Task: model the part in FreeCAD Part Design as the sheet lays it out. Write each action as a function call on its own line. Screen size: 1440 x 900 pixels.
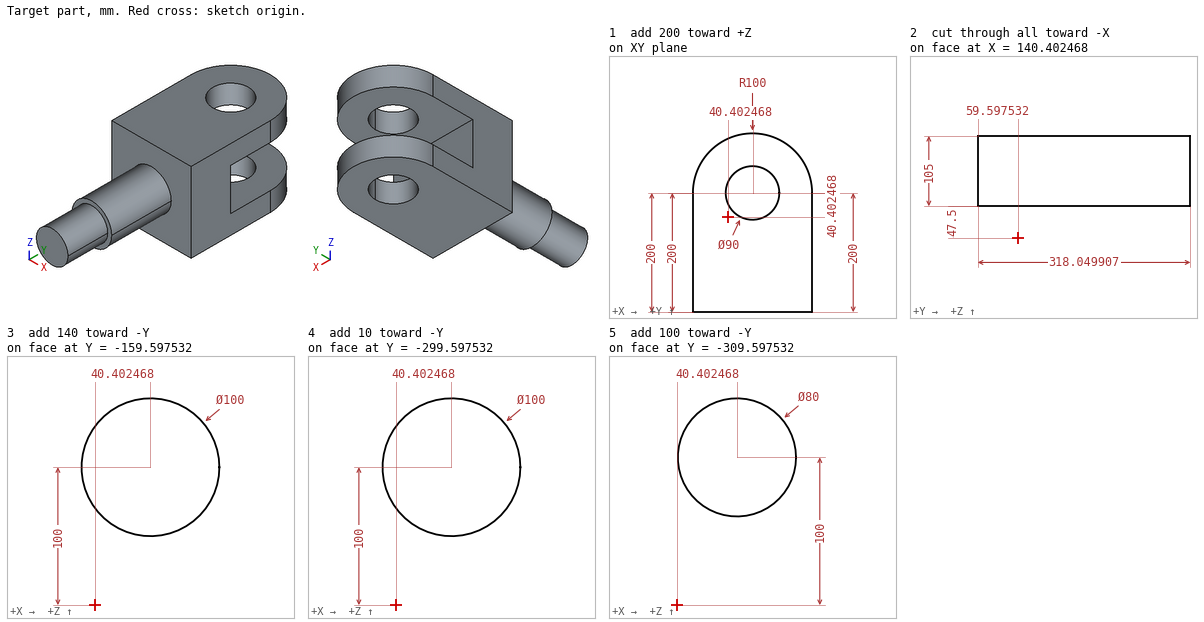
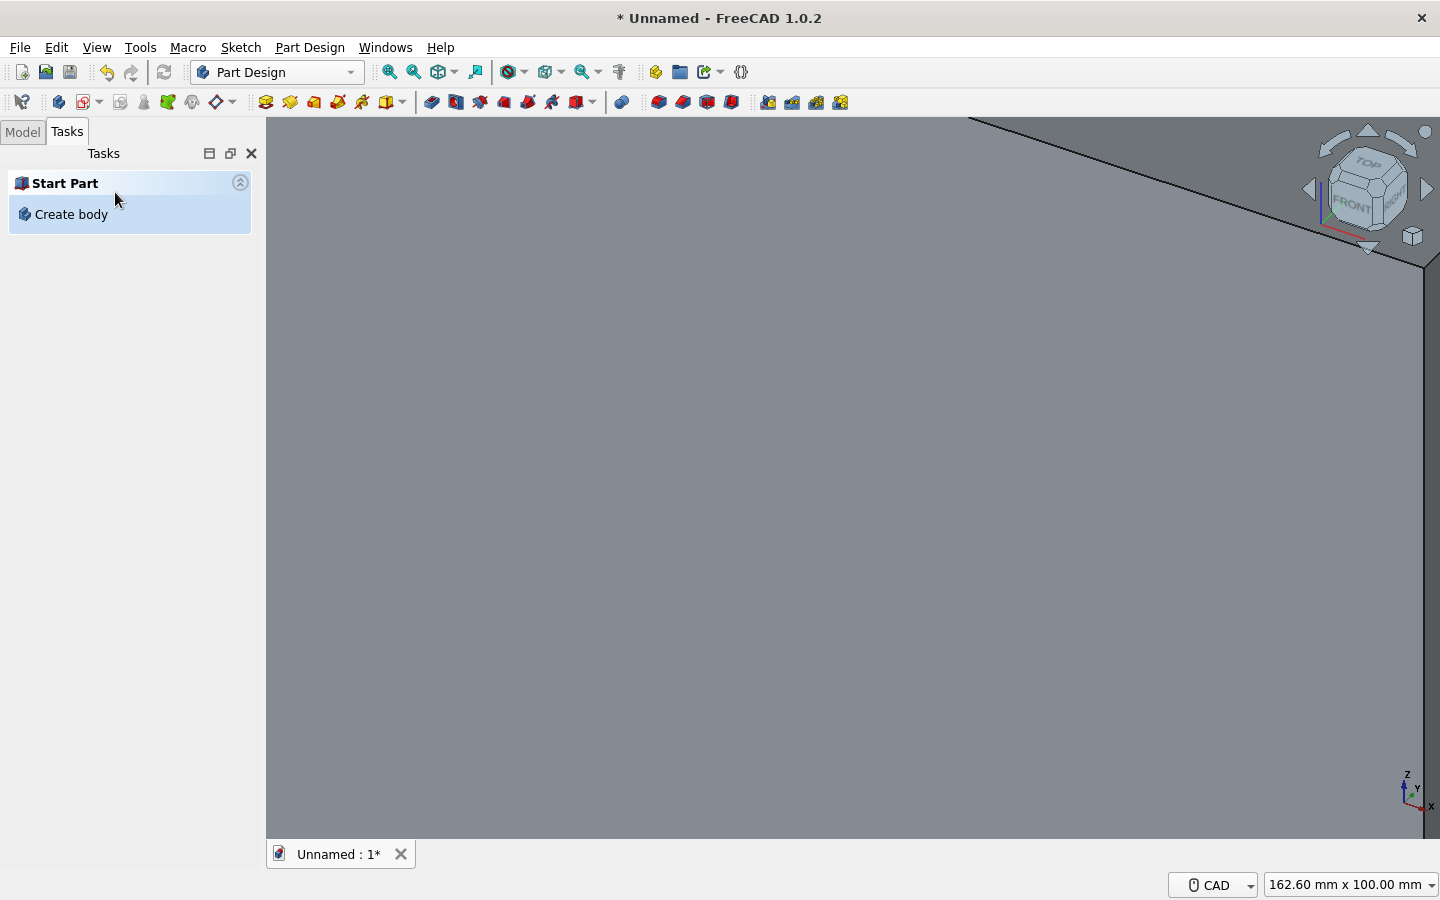
key(v)
key(f)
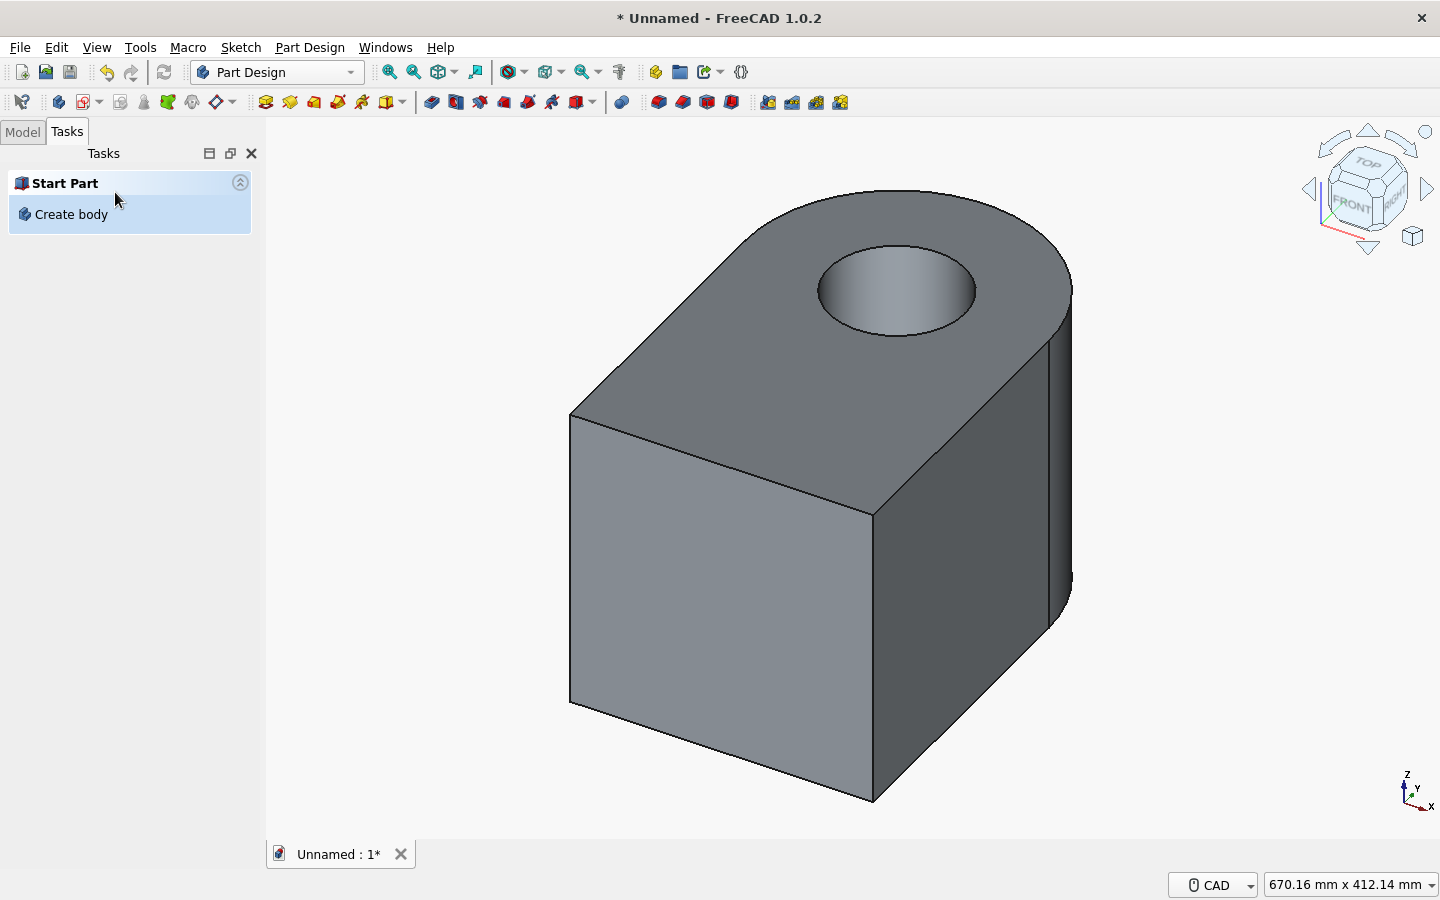
click(961, 571)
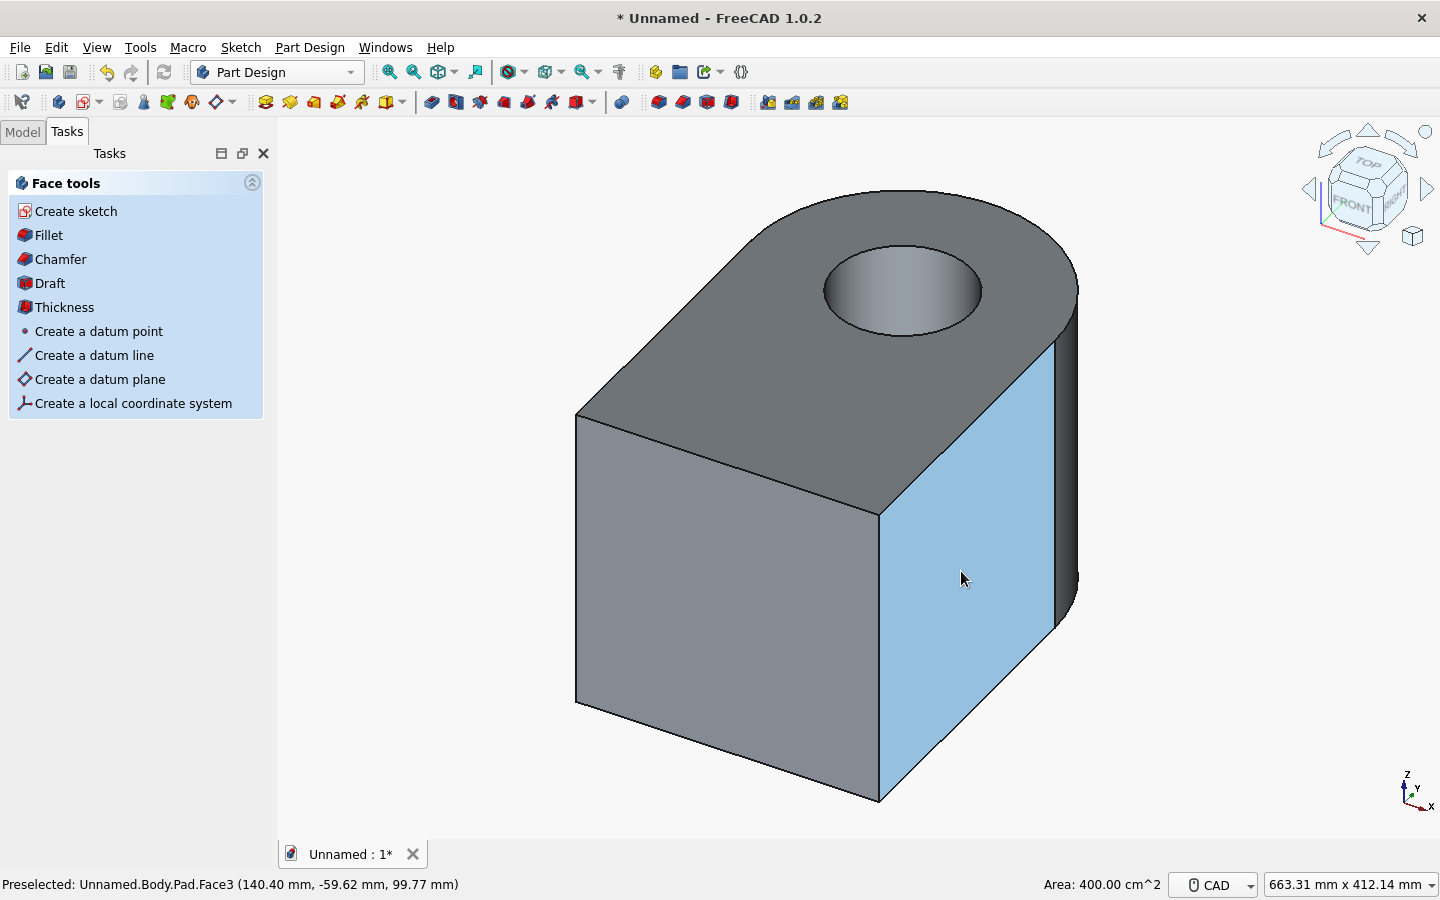
click(84, 102)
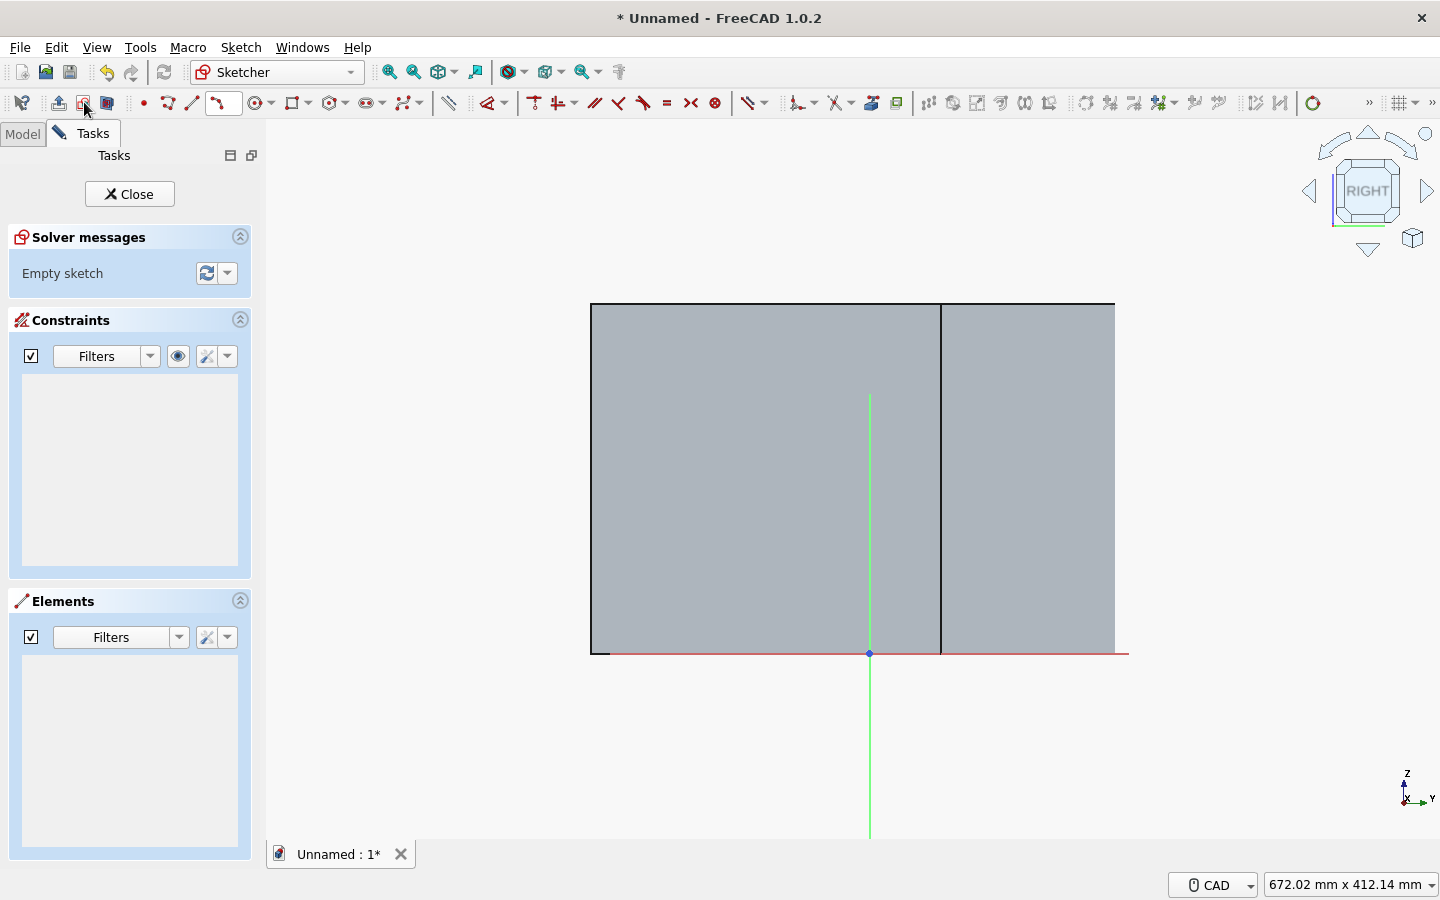
scroll(294, 292, down, 1)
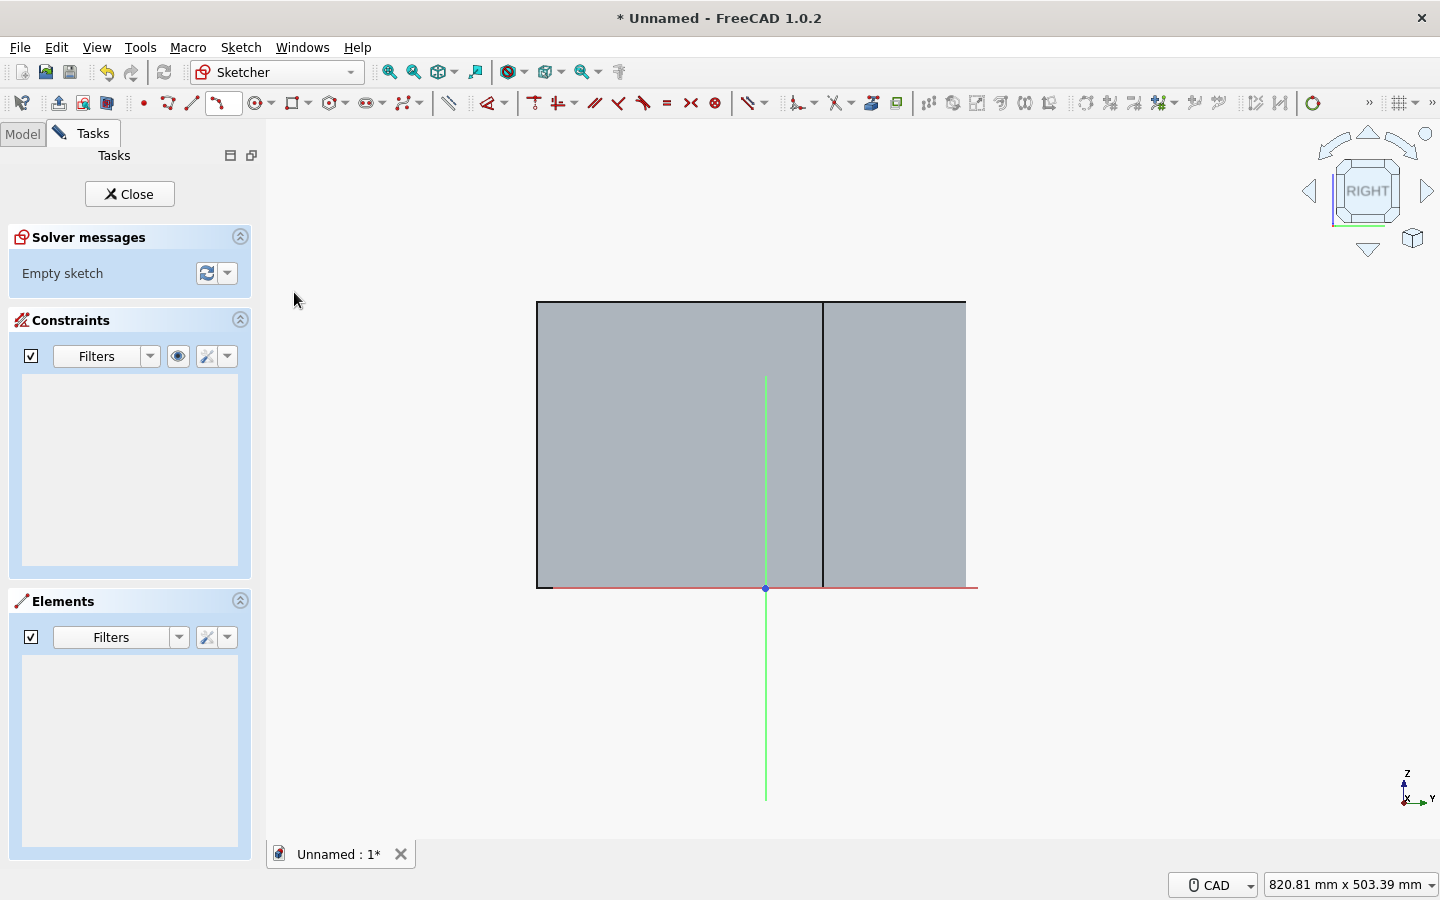
scroll(1158, 479, up, 2)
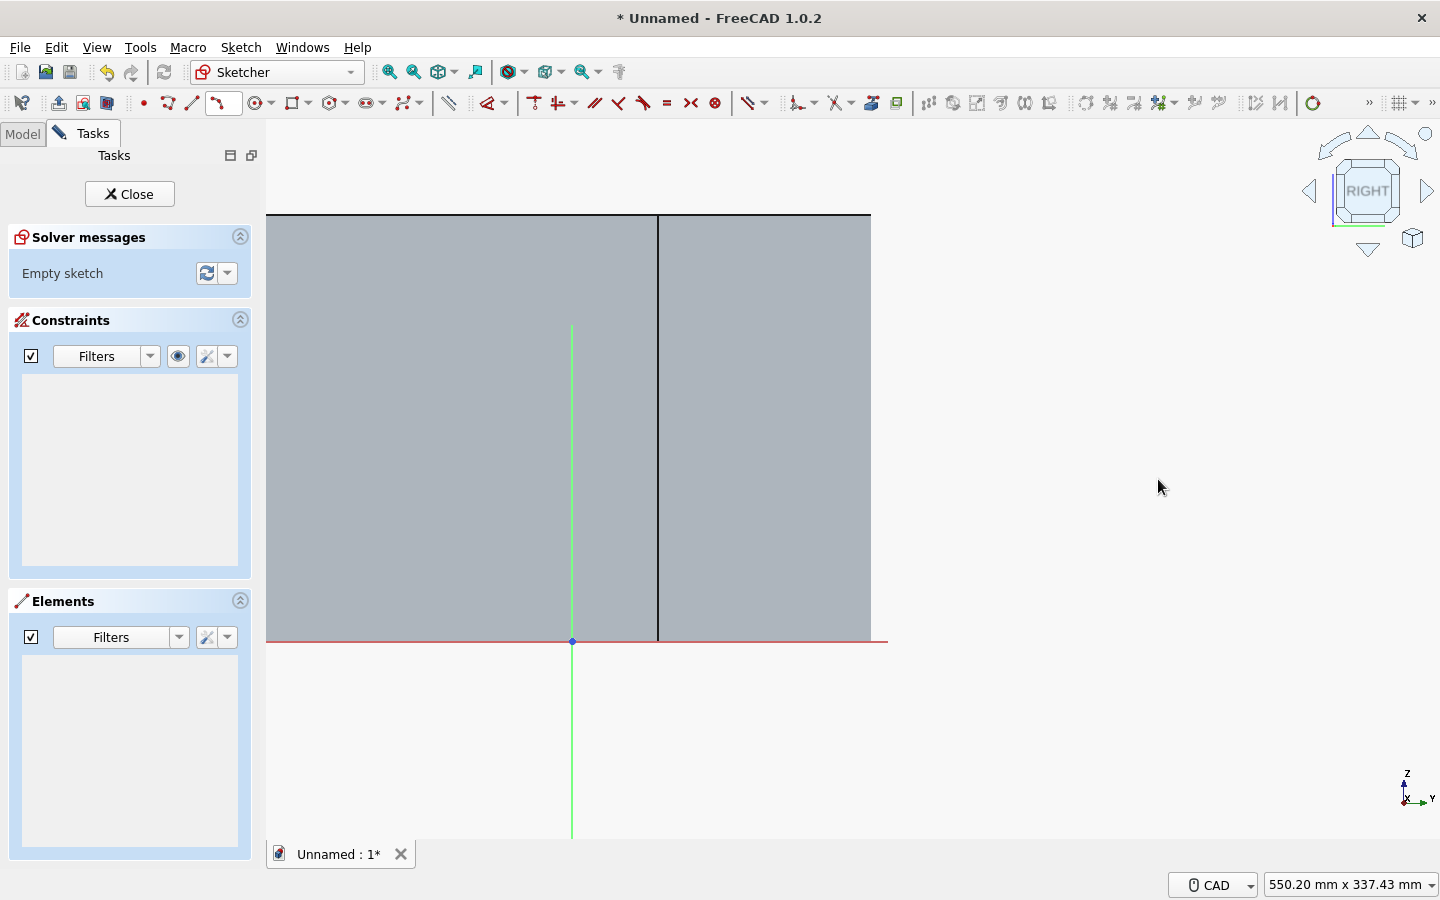
key(g)
key(r)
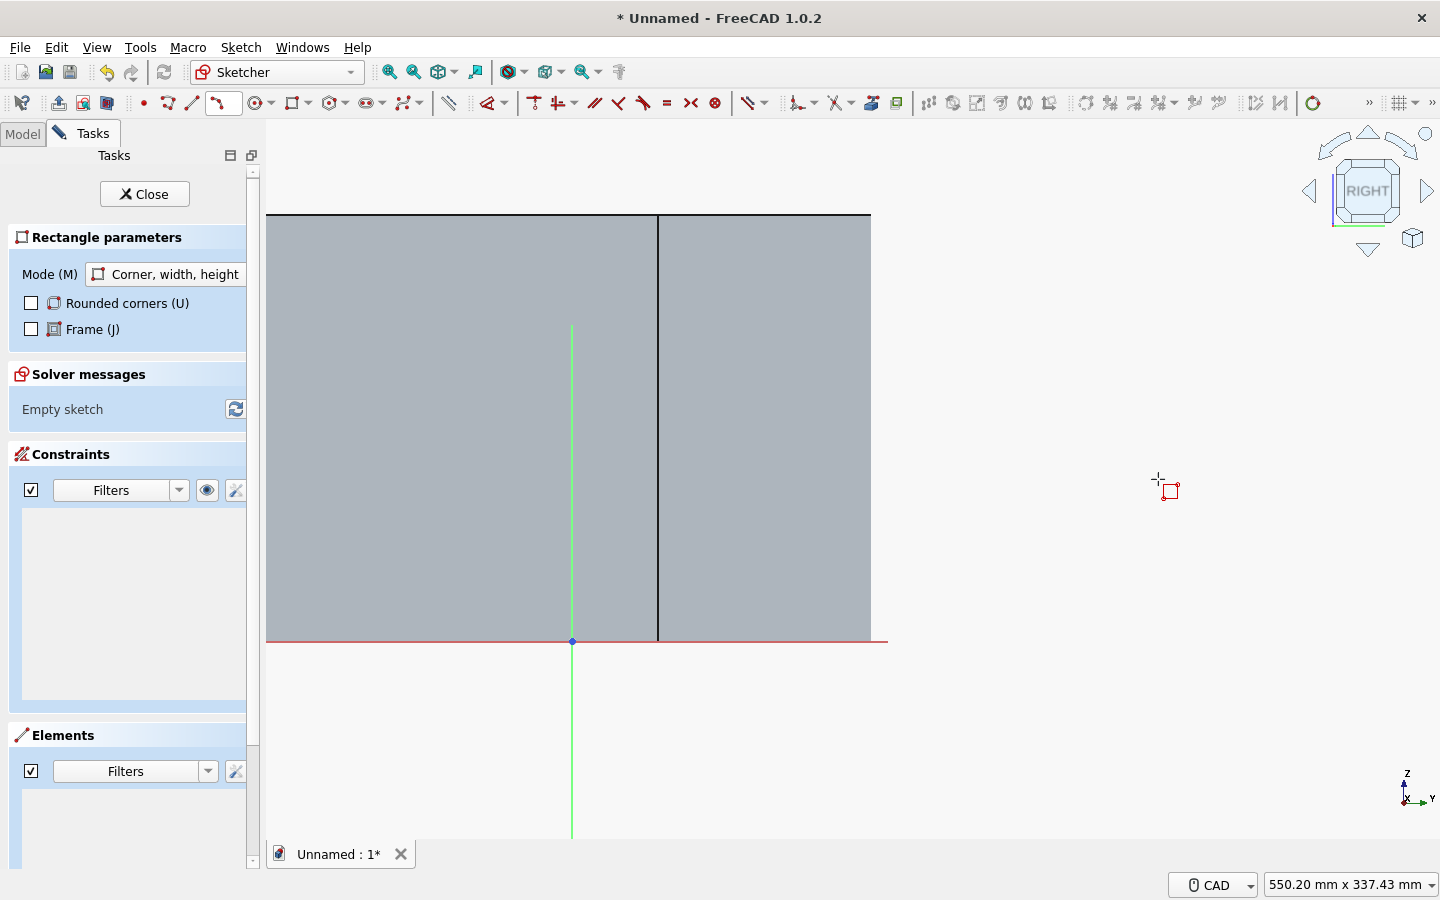
click(445, 316)
click(1124, 540)
key(Escape)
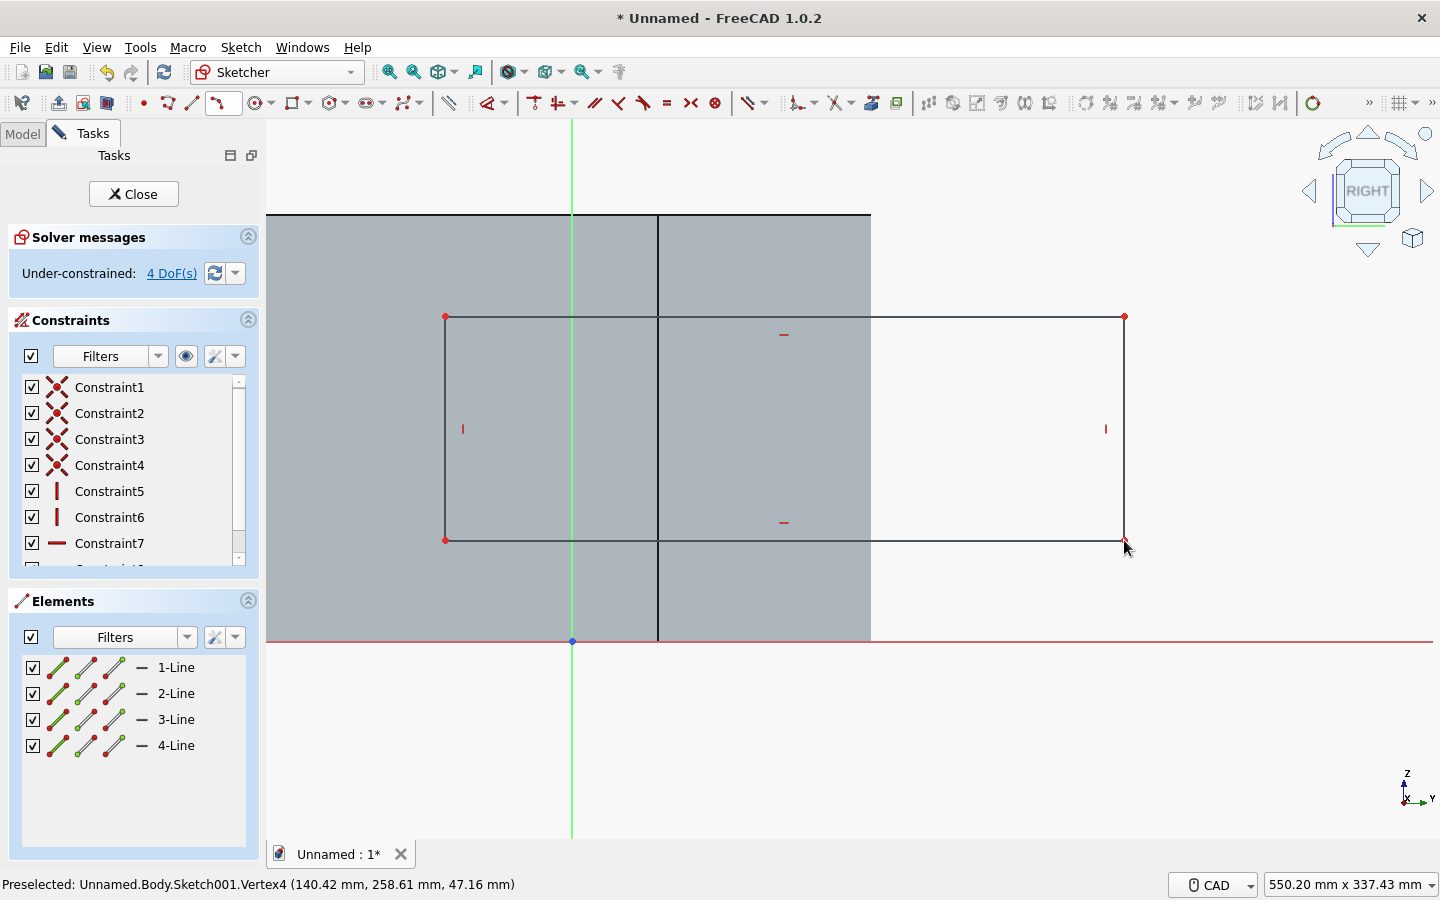
key(d)